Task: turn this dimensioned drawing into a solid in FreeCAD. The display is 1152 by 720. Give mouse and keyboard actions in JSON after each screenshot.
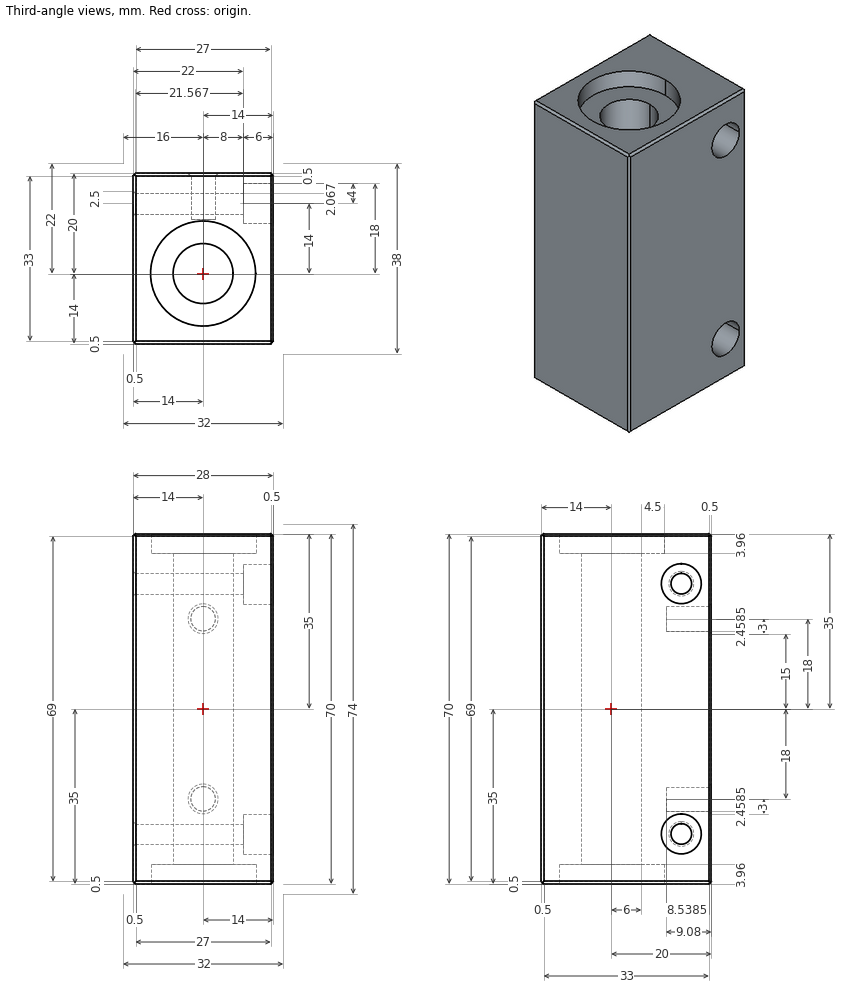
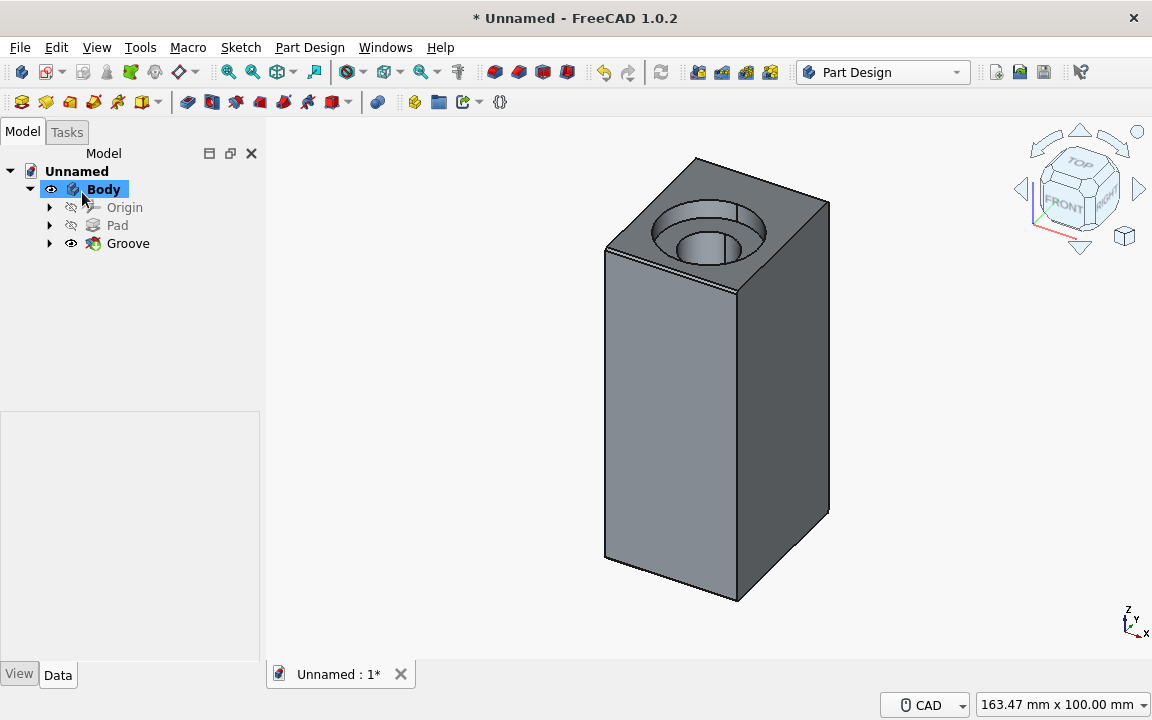
{"action": "left_click", "coordinate": [50, 207]}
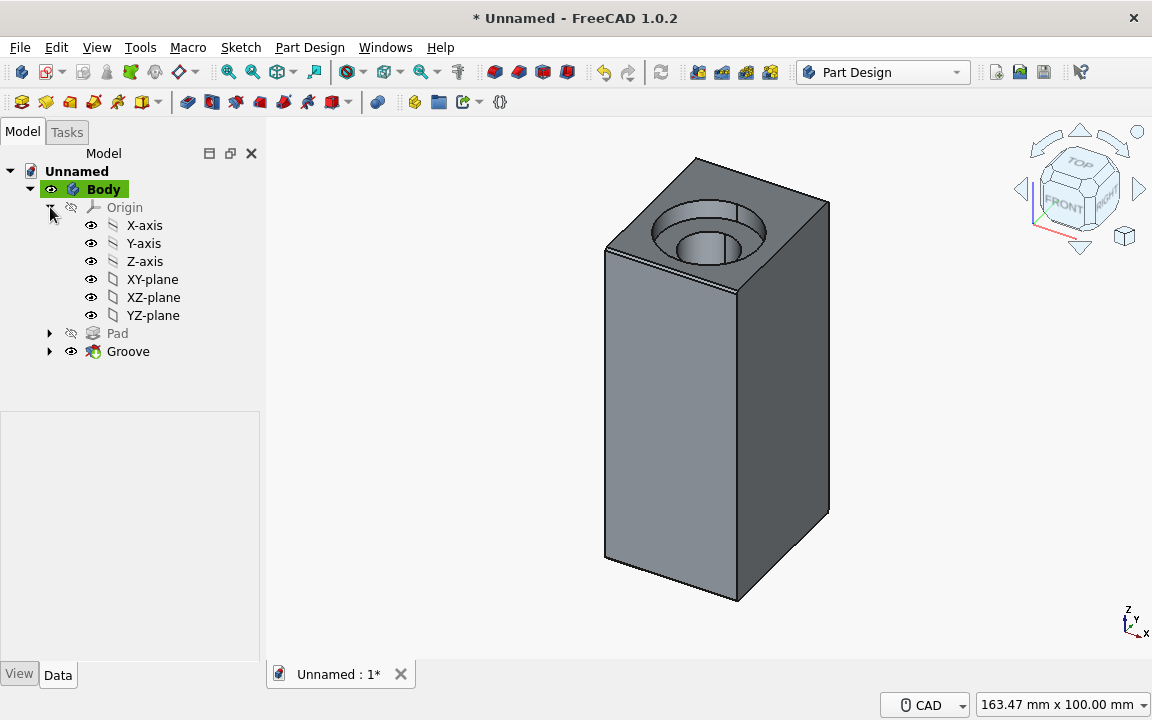
{"action": "left_click", "coordinate": [136, 279]}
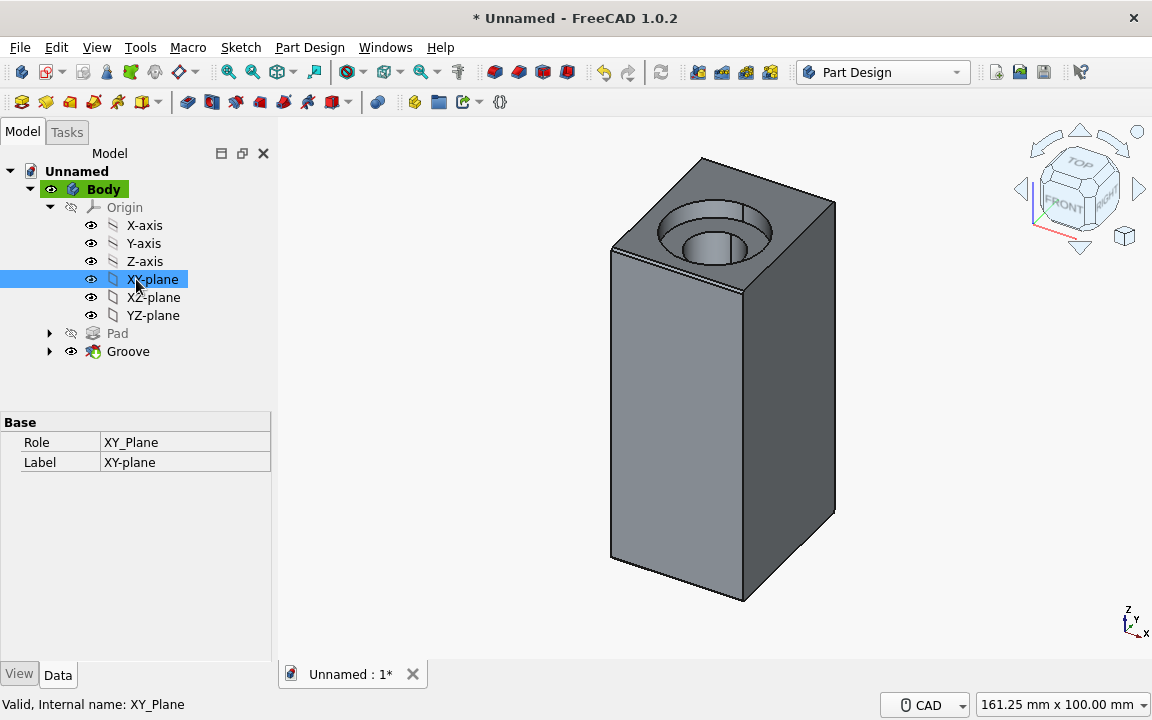
{"action": "left_click", "coordinate": [180, 72]}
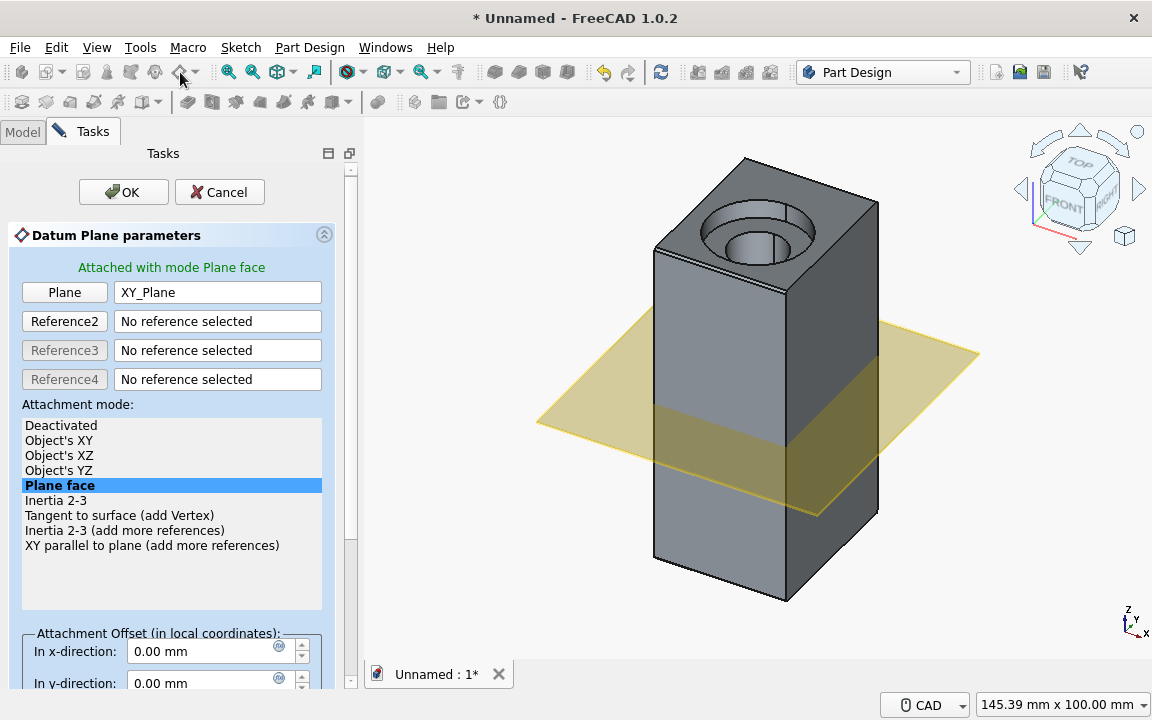
{"action": "scroll", "coordinate": [351, 426], "scroll_direction": "down", "scroll_amount": 2}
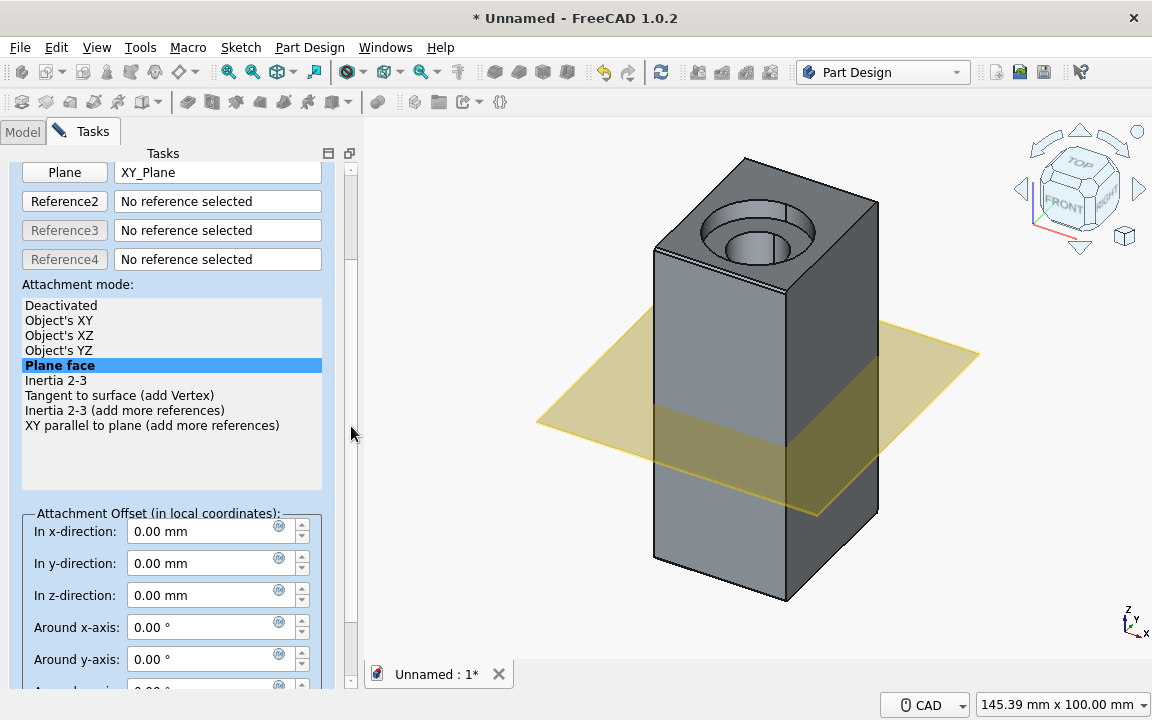
{"action": "triple_click", "coordinate": [210, 595]}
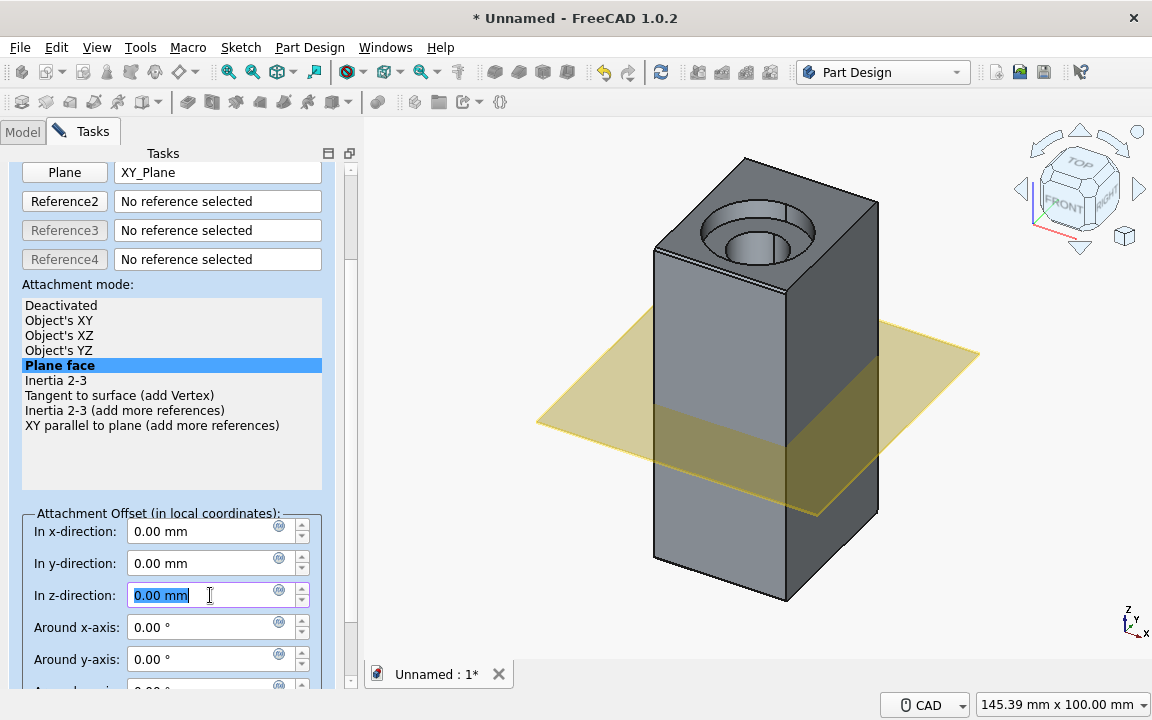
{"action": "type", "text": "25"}
{"action": "key", "text": "Tab"}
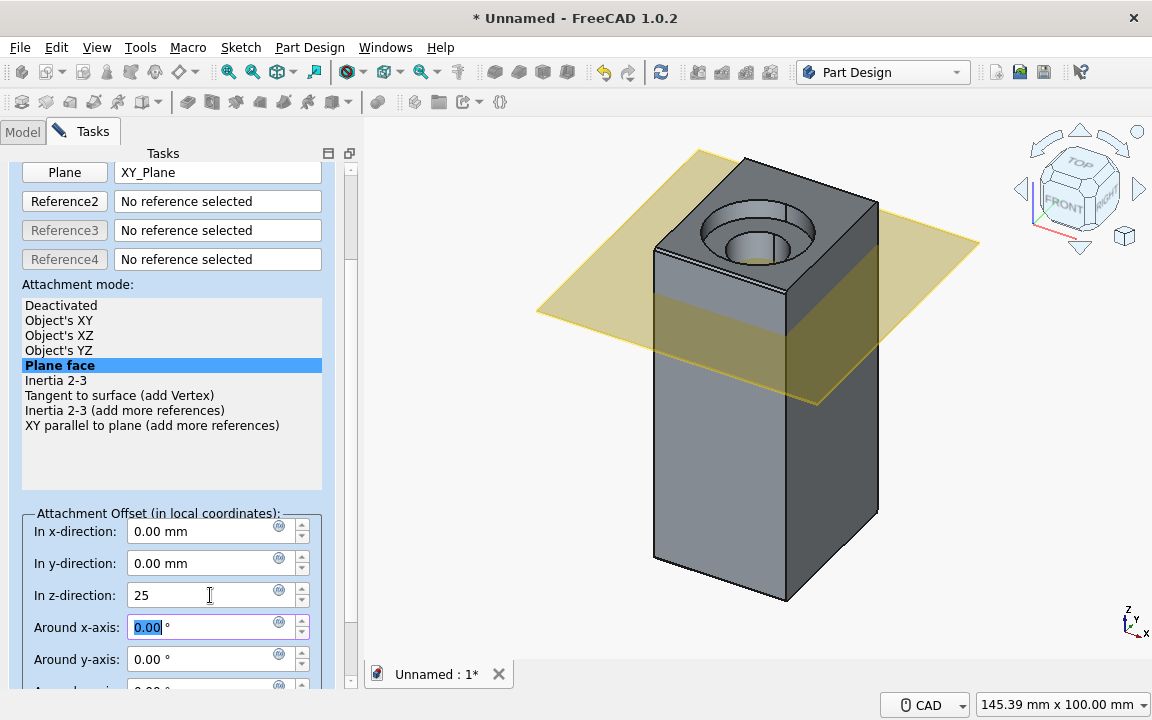
{"action": "scroll", "coordinate": [351, 426], "scroll_direction": "up", "scroll_amount": 3}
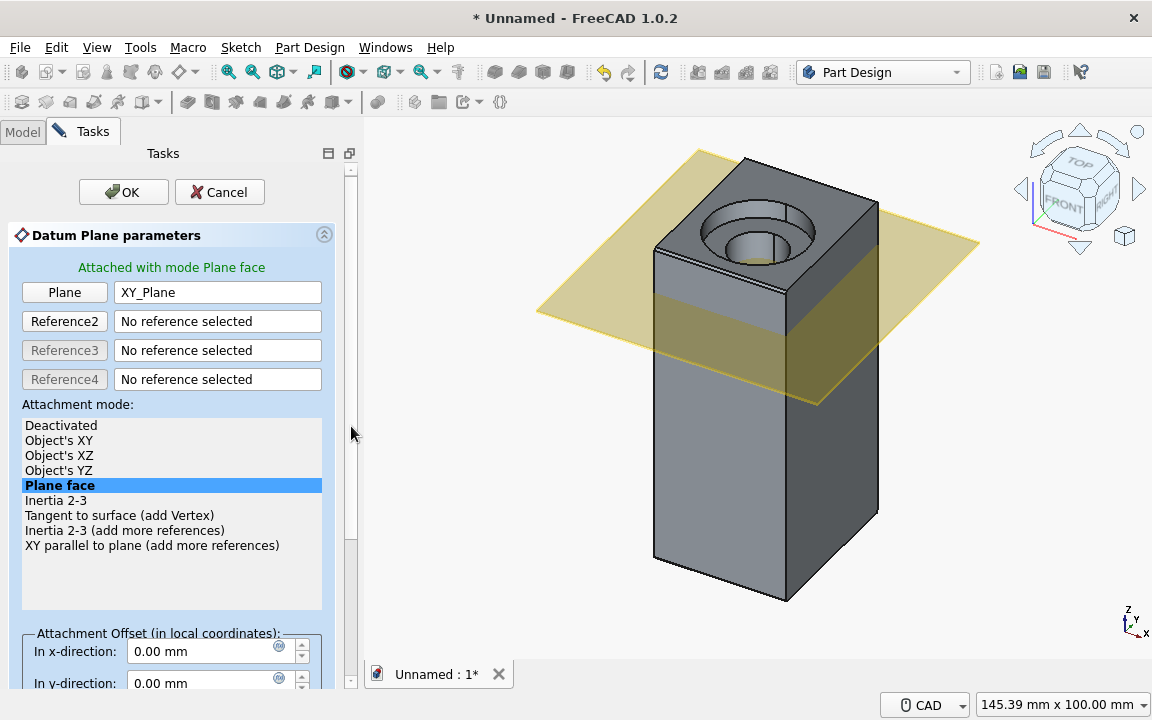
{"action": "left_click", "coordinate": [124, 192]}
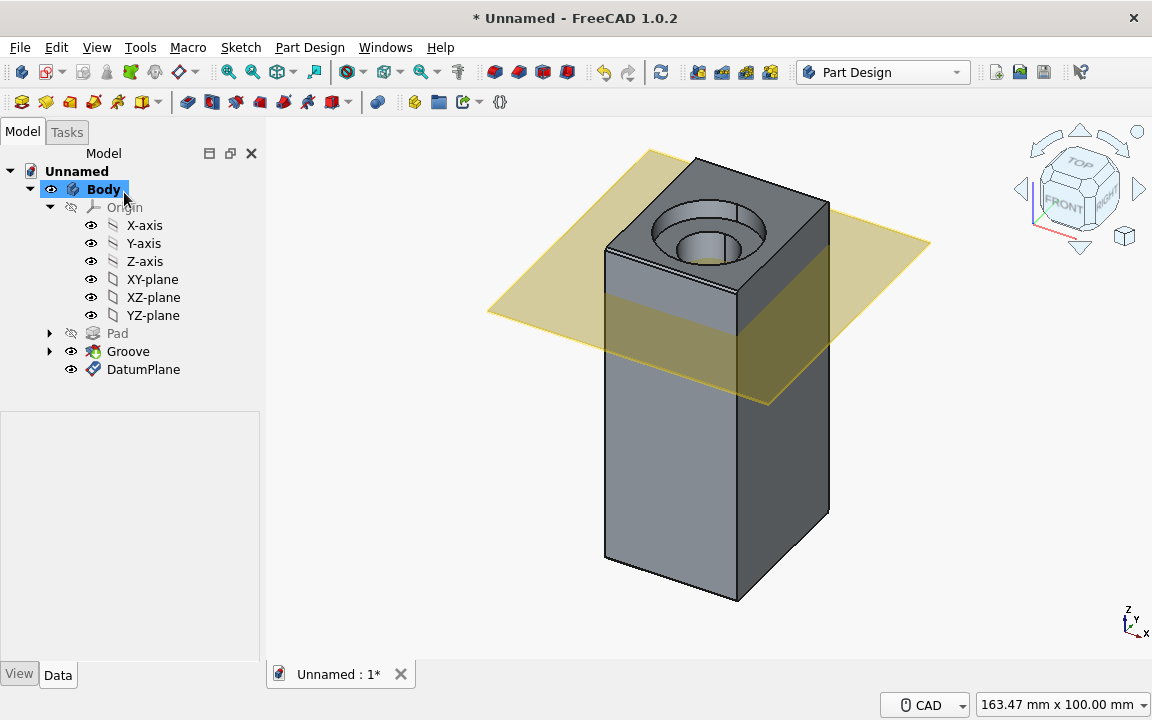
{"action": "left_click", "coordinate": [116, 369]}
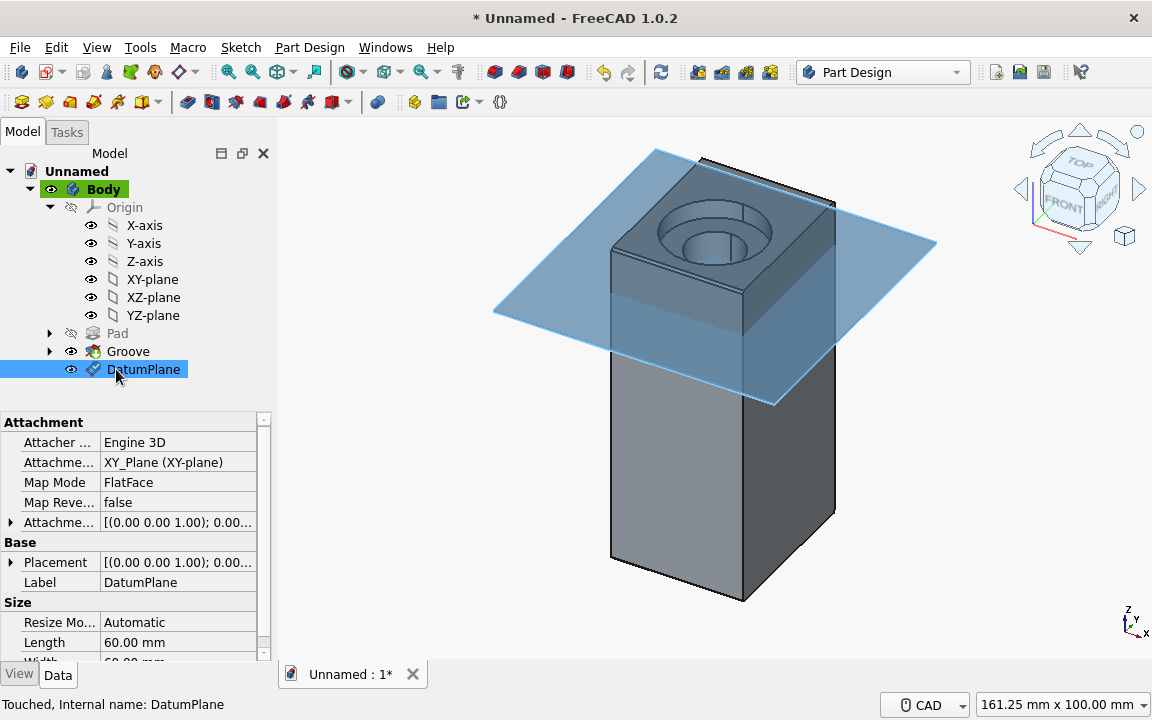
{"action": "left_click", "coordinate": [46, 72]}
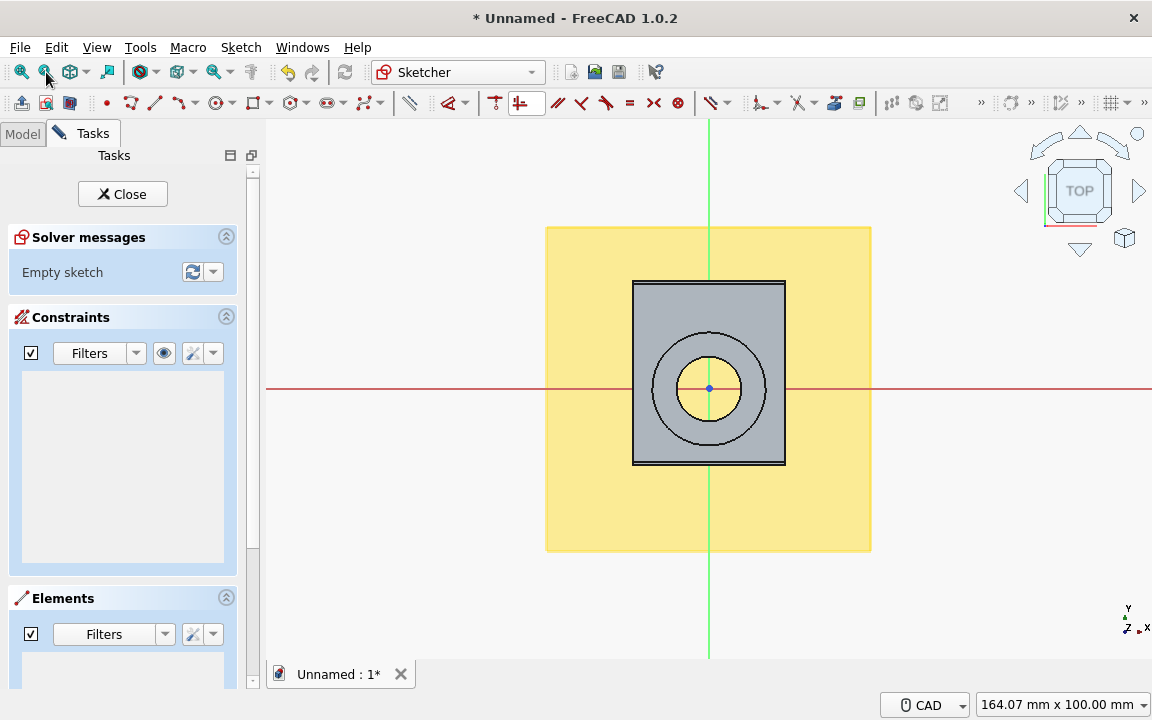
{"action": "left_click", "coordinate": [70, 104]}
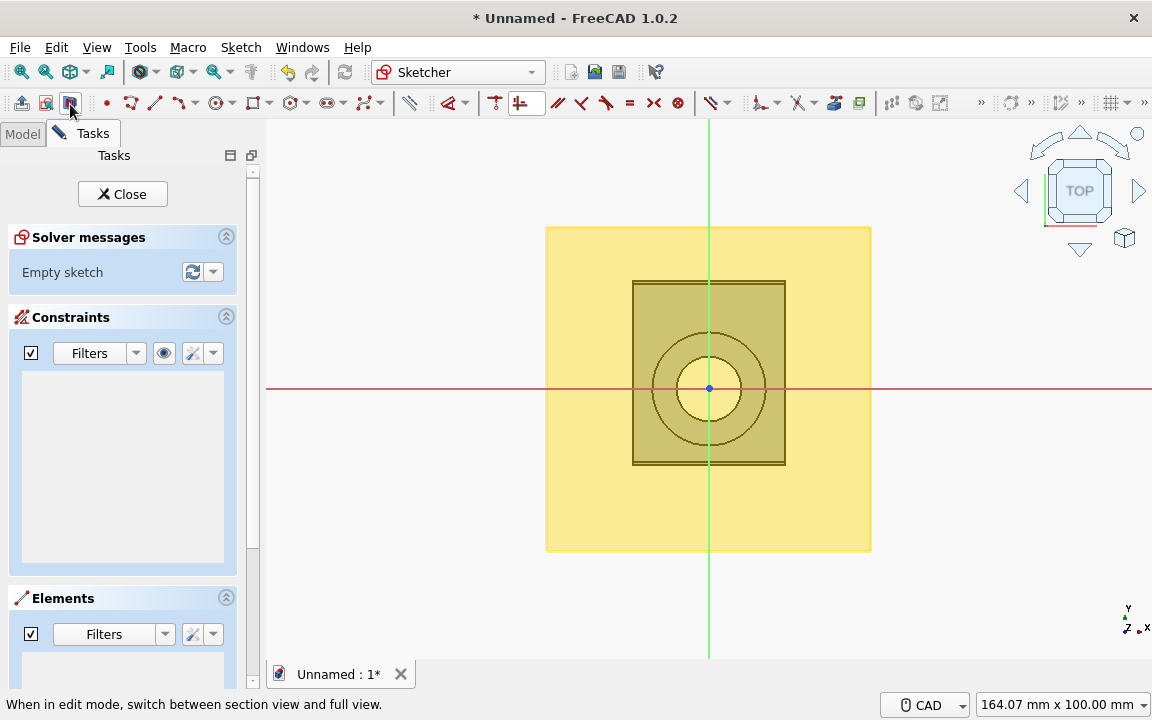
{"action": "scroll", "coordinate": [793, 319], "scroll_direction": "up", "scroll_amount": 6}